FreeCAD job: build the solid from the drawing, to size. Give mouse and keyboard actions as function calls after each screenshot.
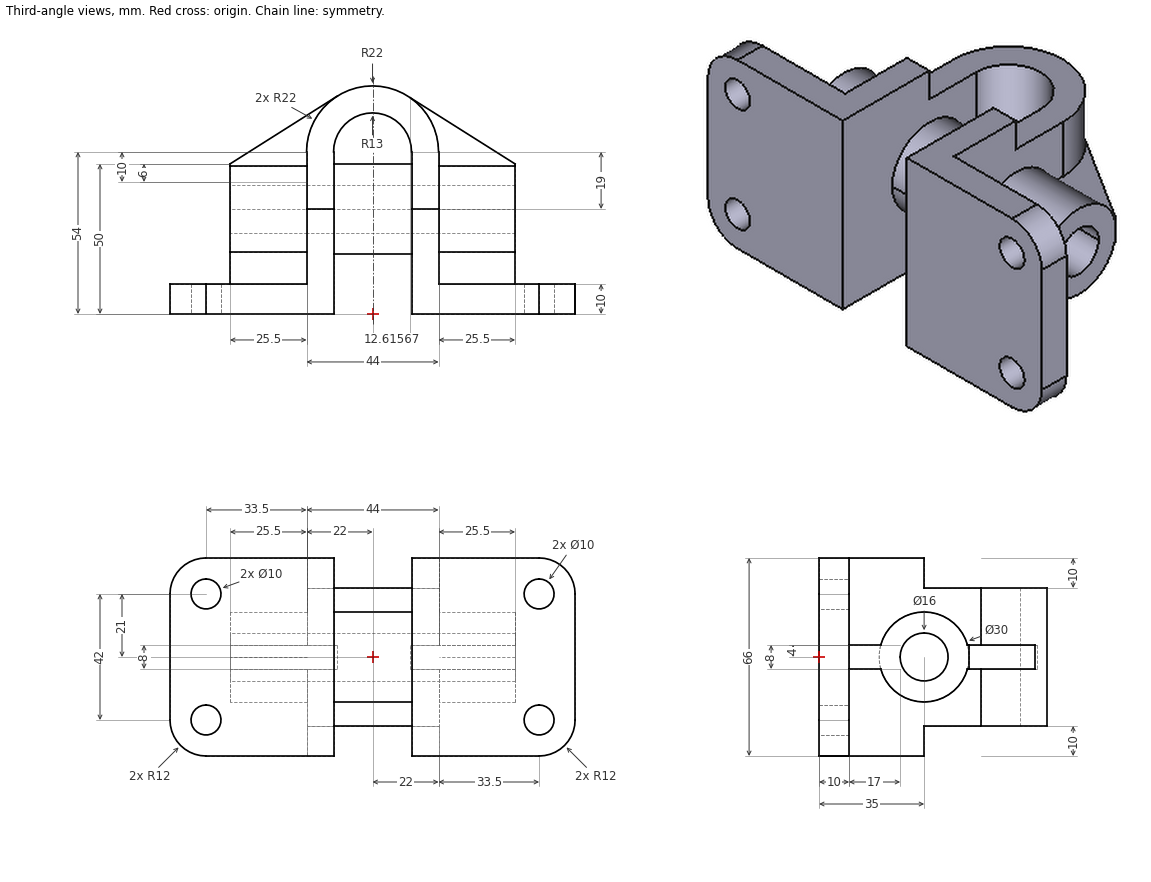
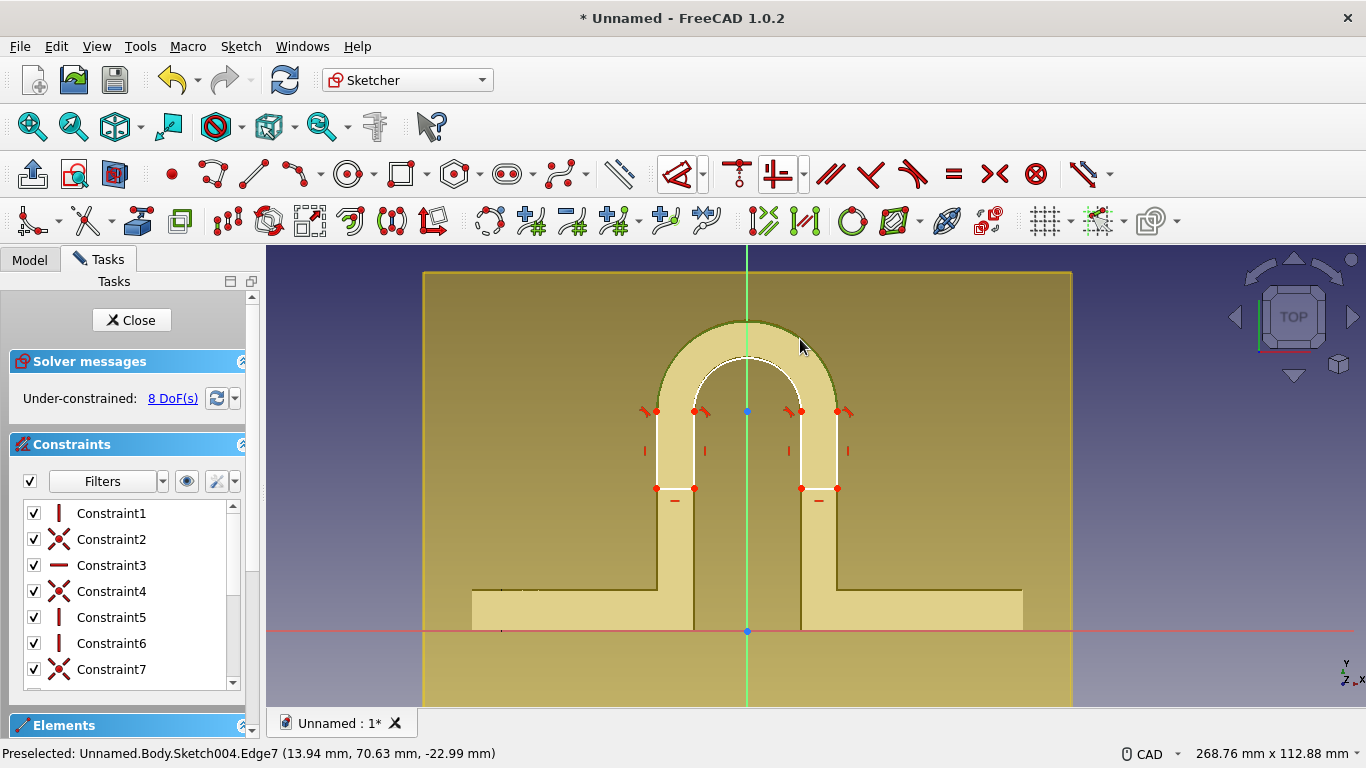
click(779, 368)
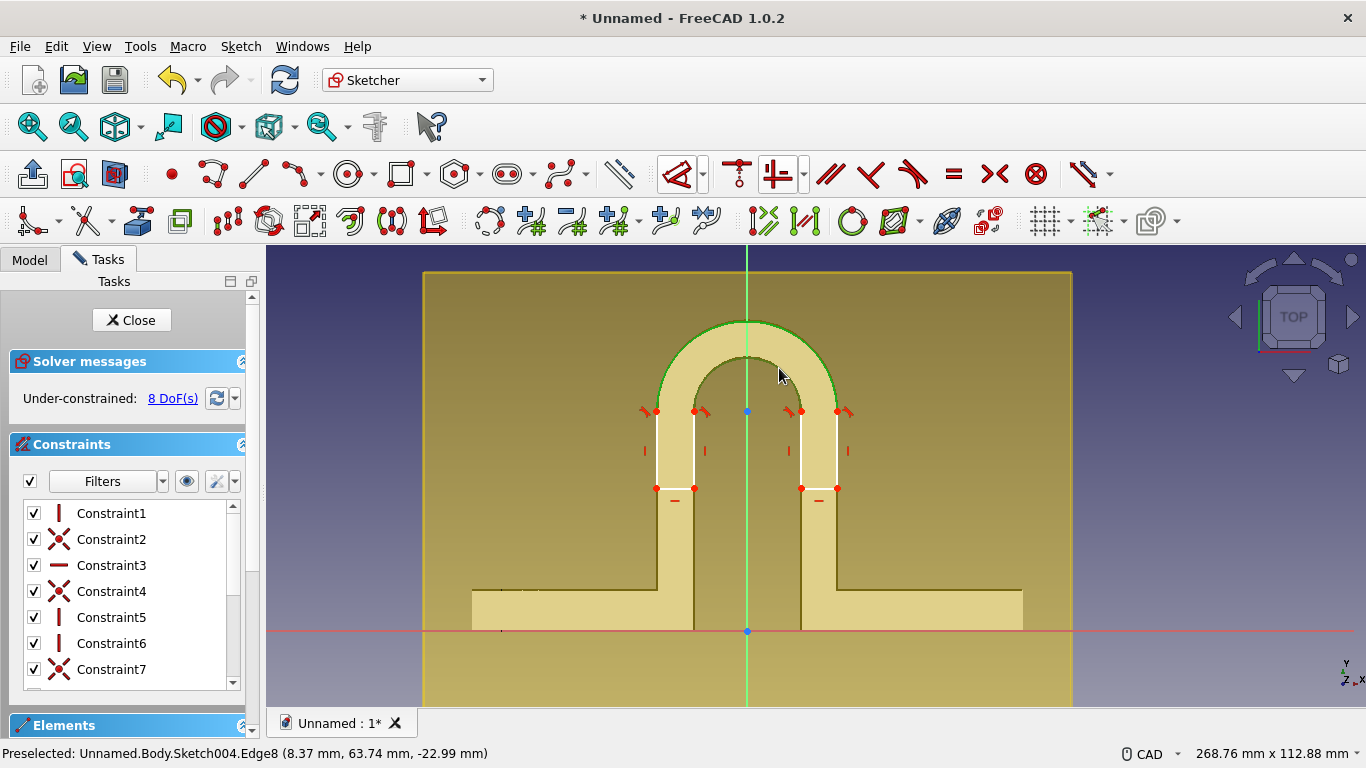
click(737, 174)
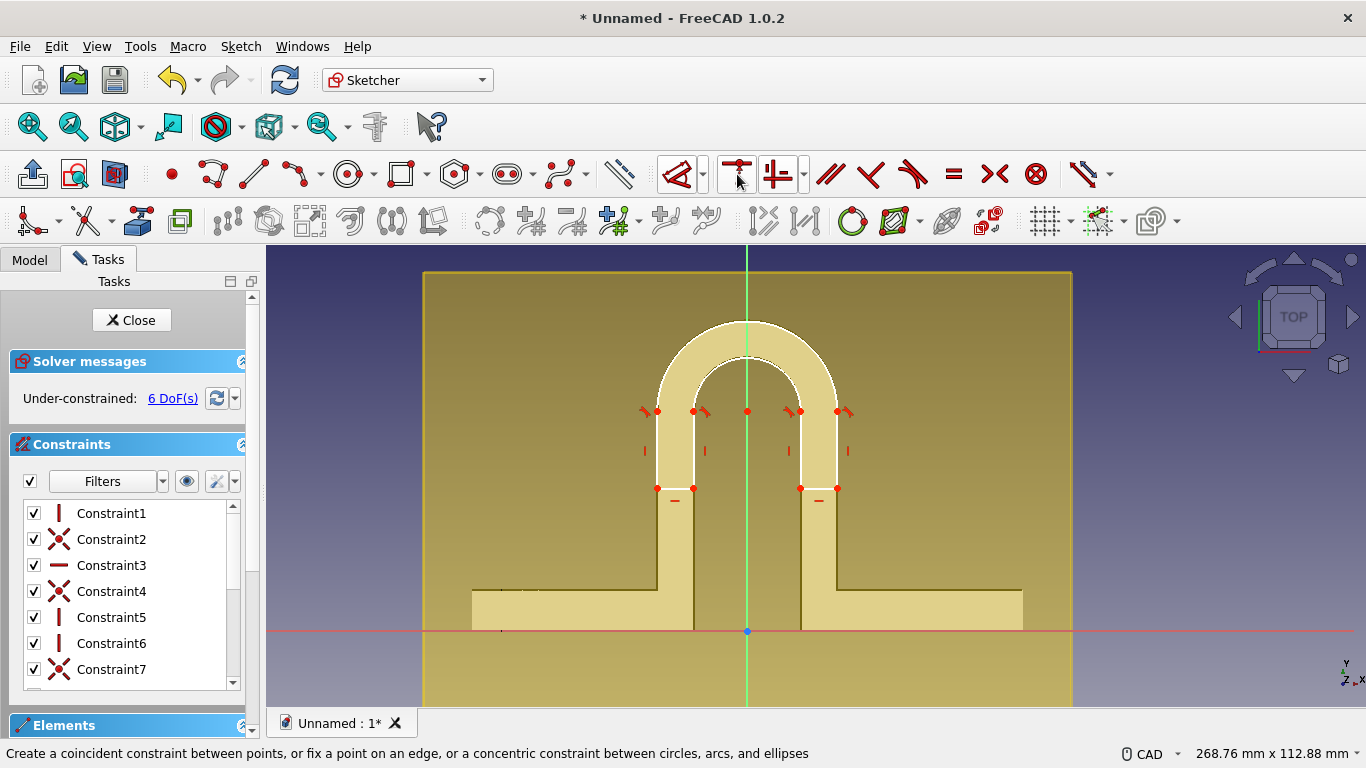
click(747, 412)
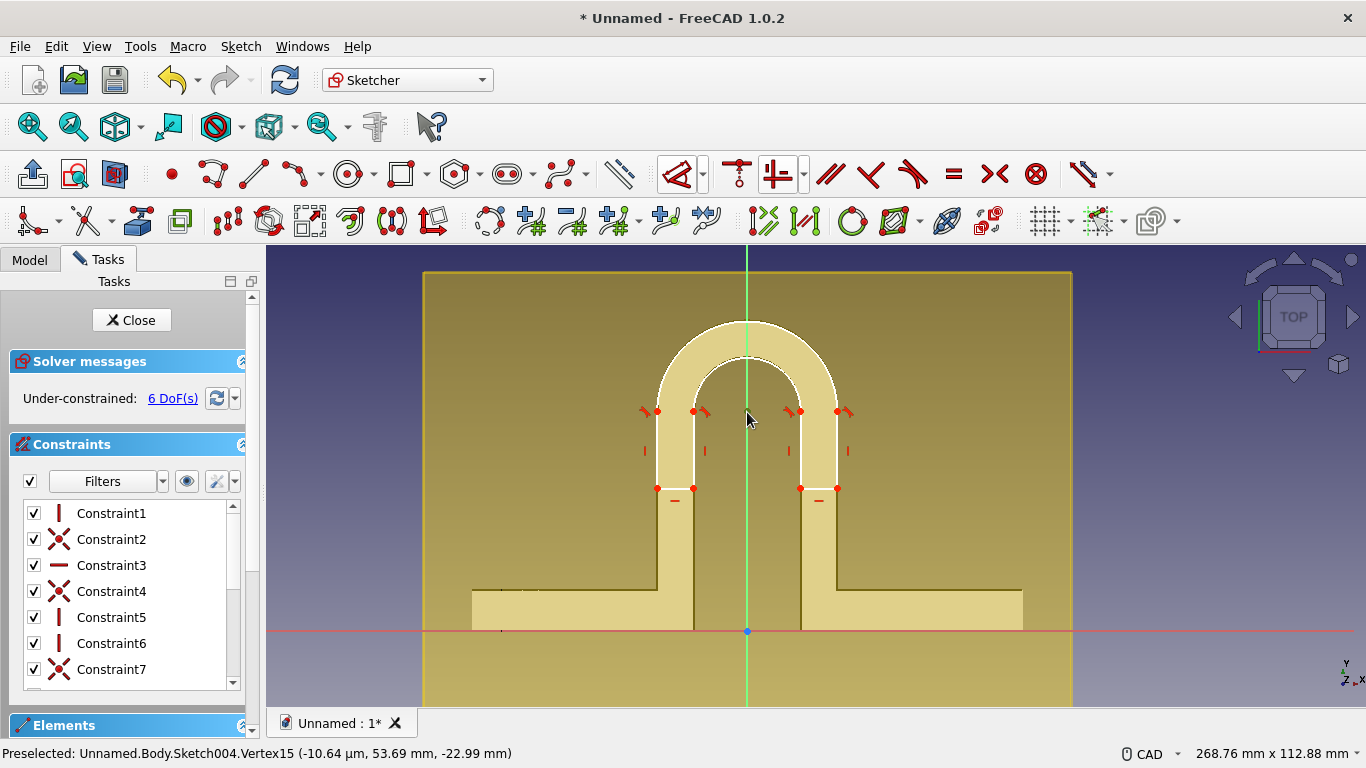
click(747, 592)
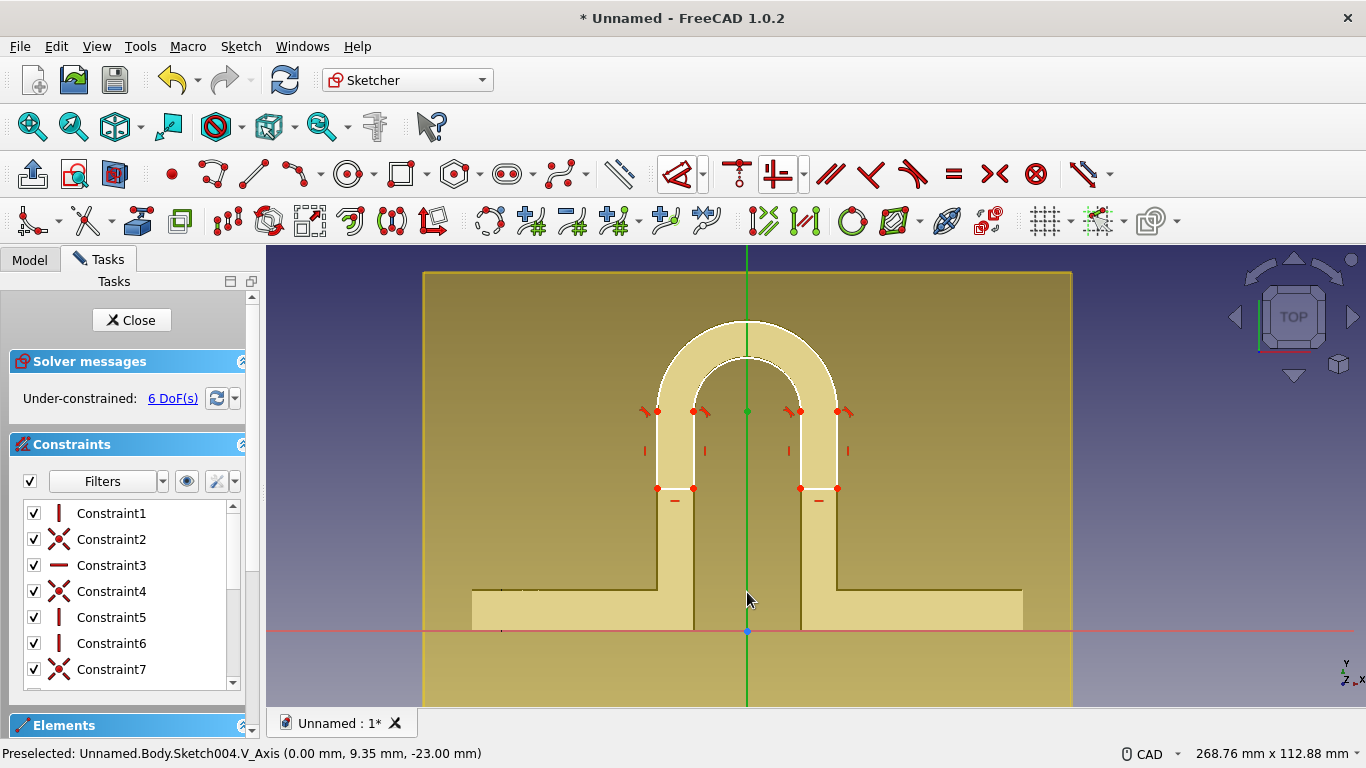
click(737, 174)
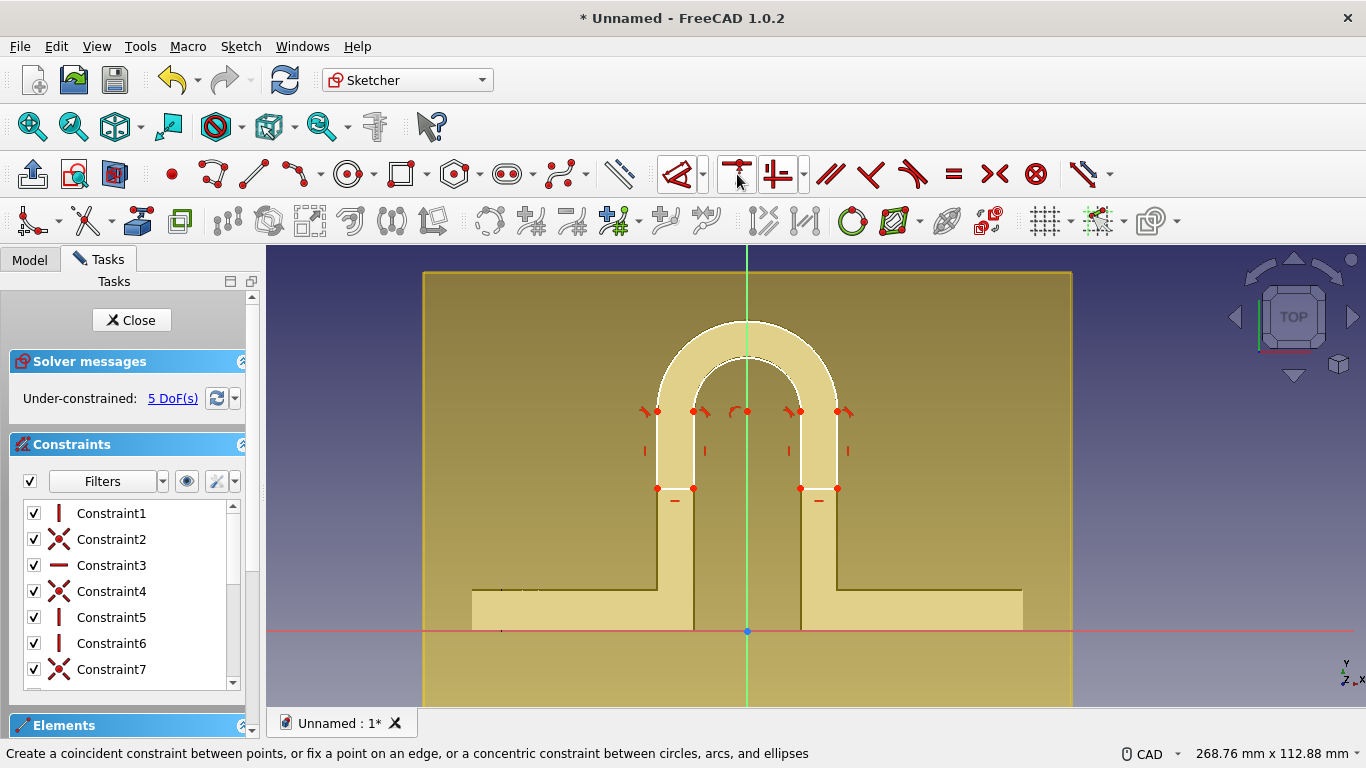
click(800, 339)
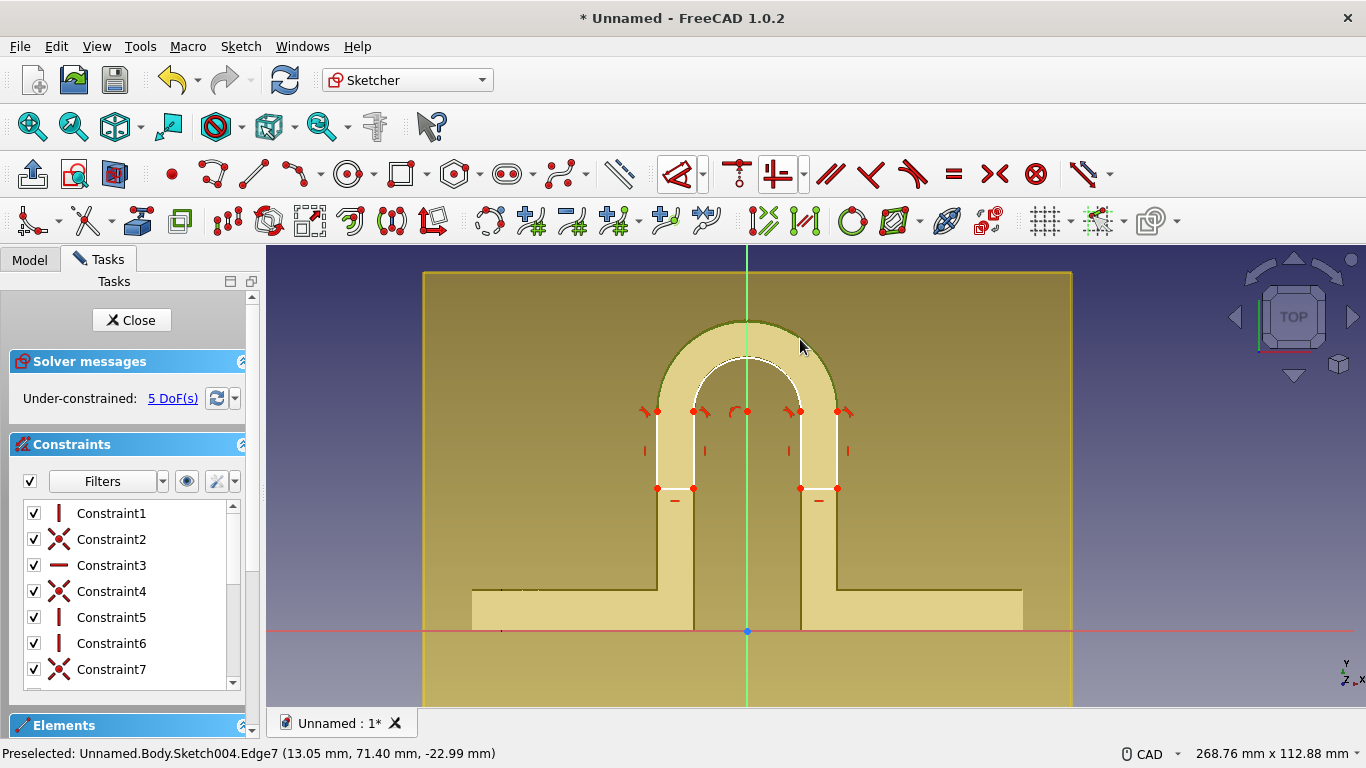
key(k)
key(r)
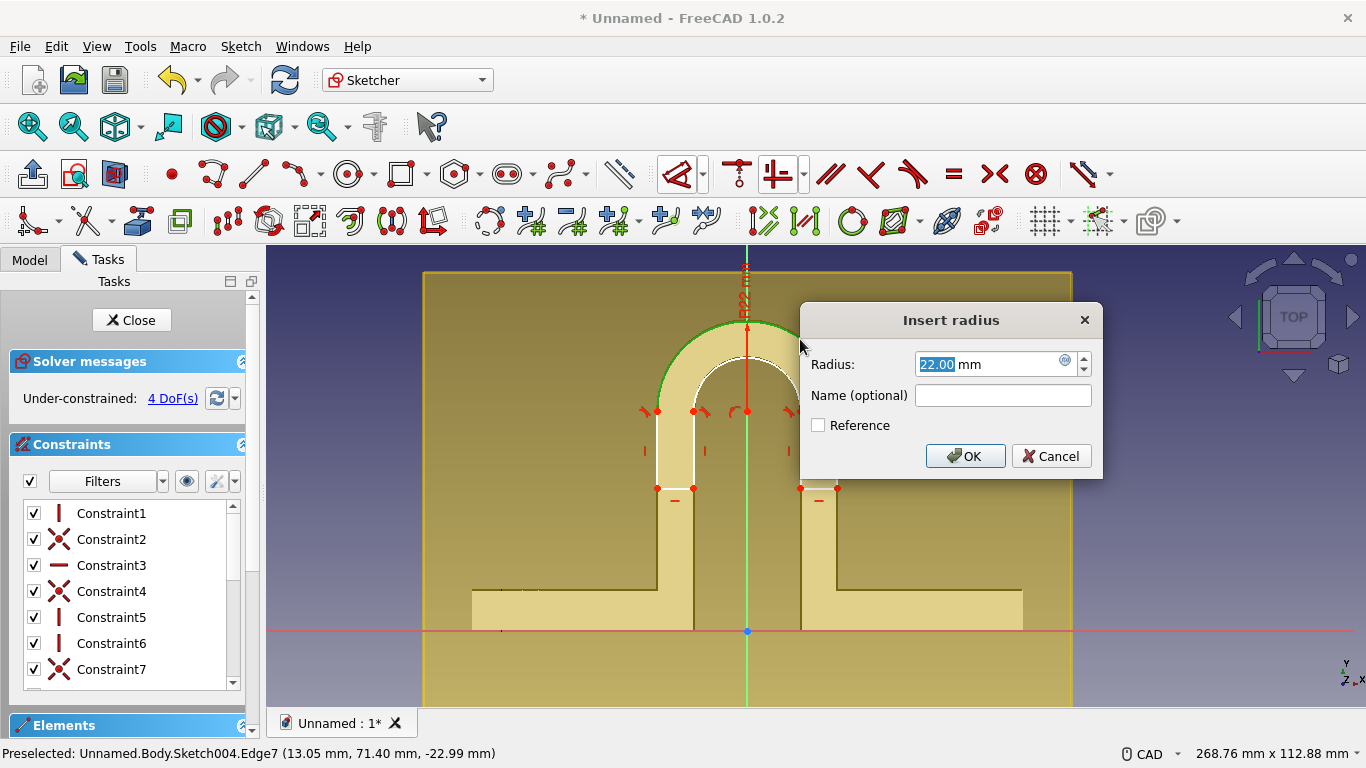
text(22)
key(Return)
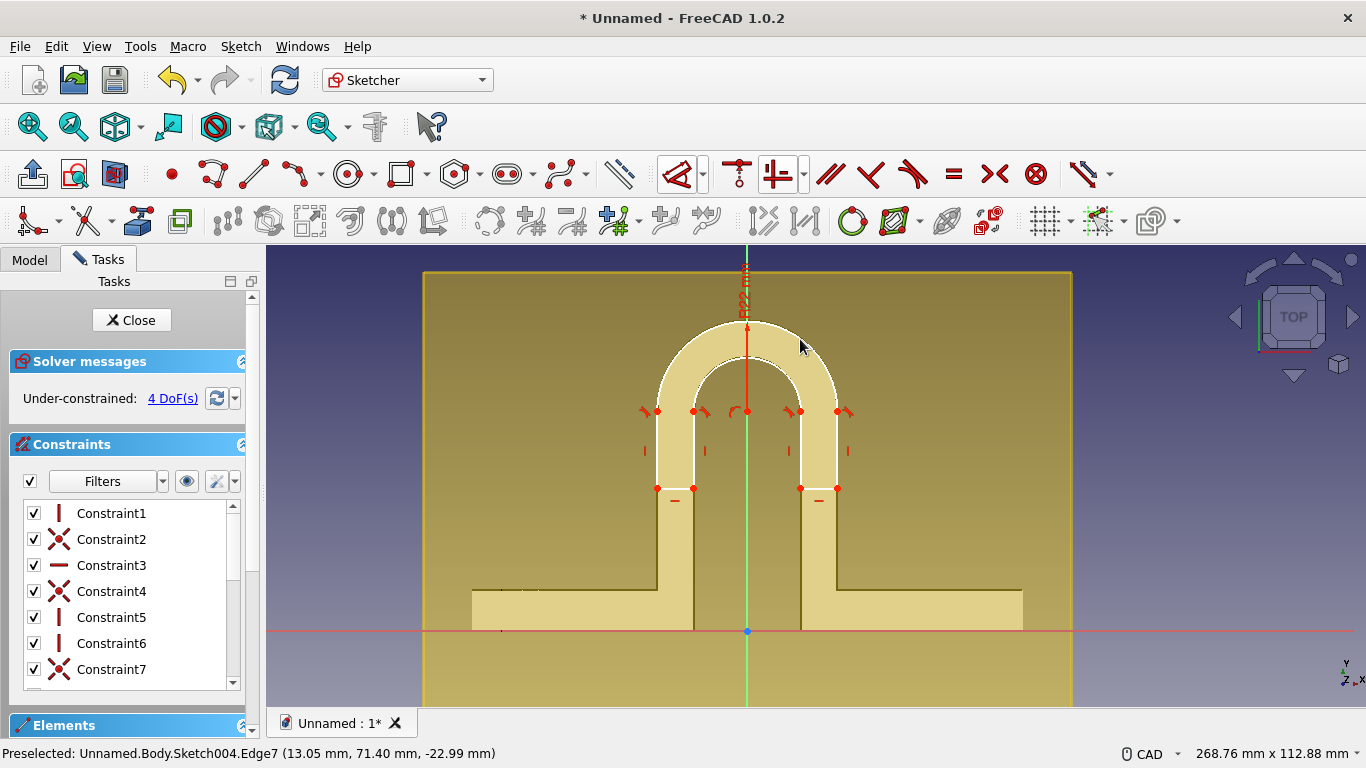
click(779, 368)